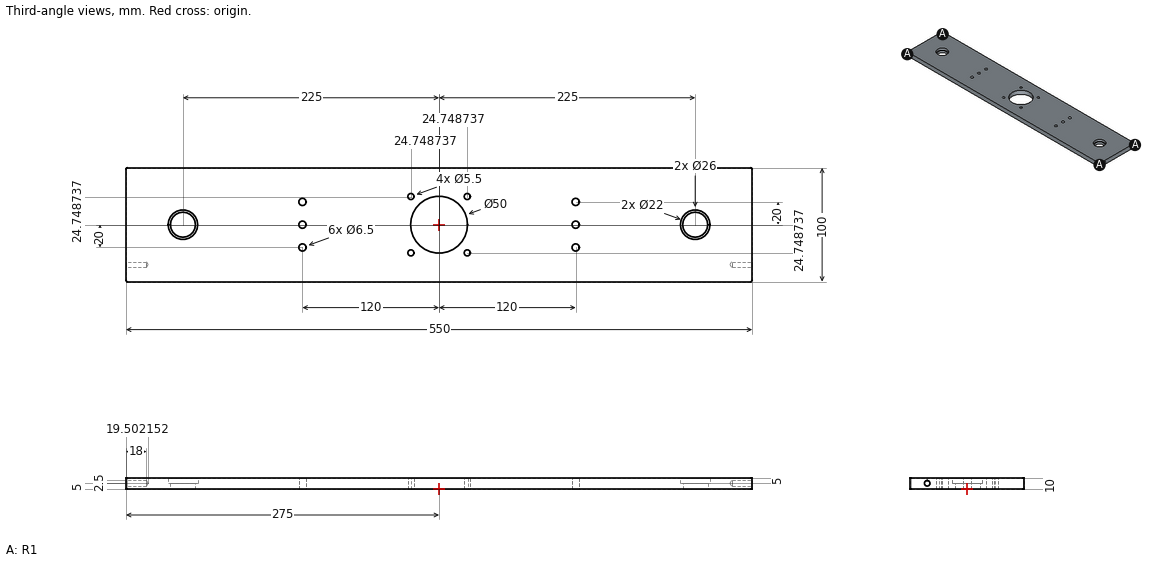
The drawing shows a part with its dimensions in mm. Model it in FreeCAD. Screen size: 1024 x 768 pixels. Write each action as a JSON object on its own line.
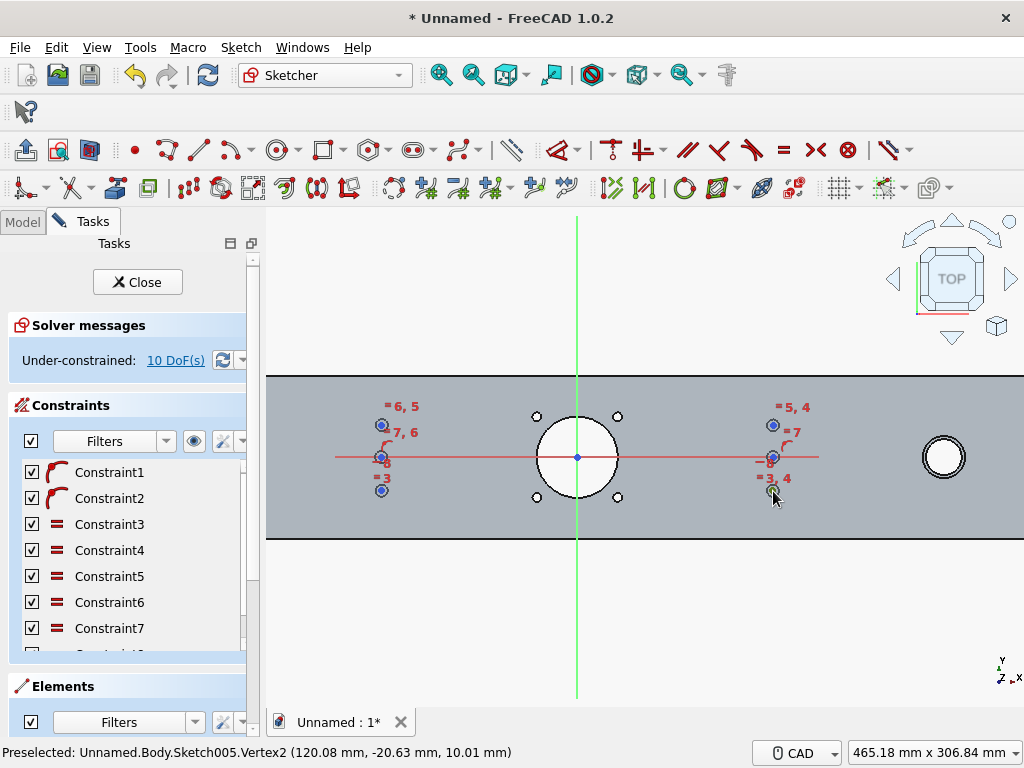
{"action": "left_click", "coordinate": [773, 425]}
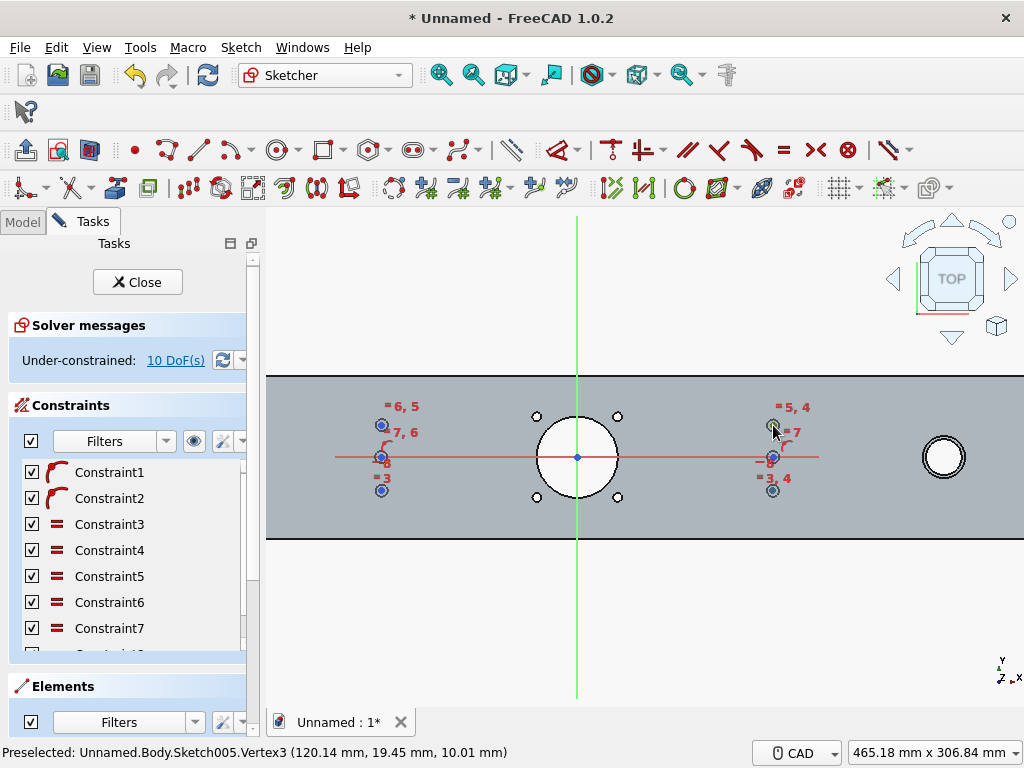
{"action": "left_click", "coordinate": [666, 150]}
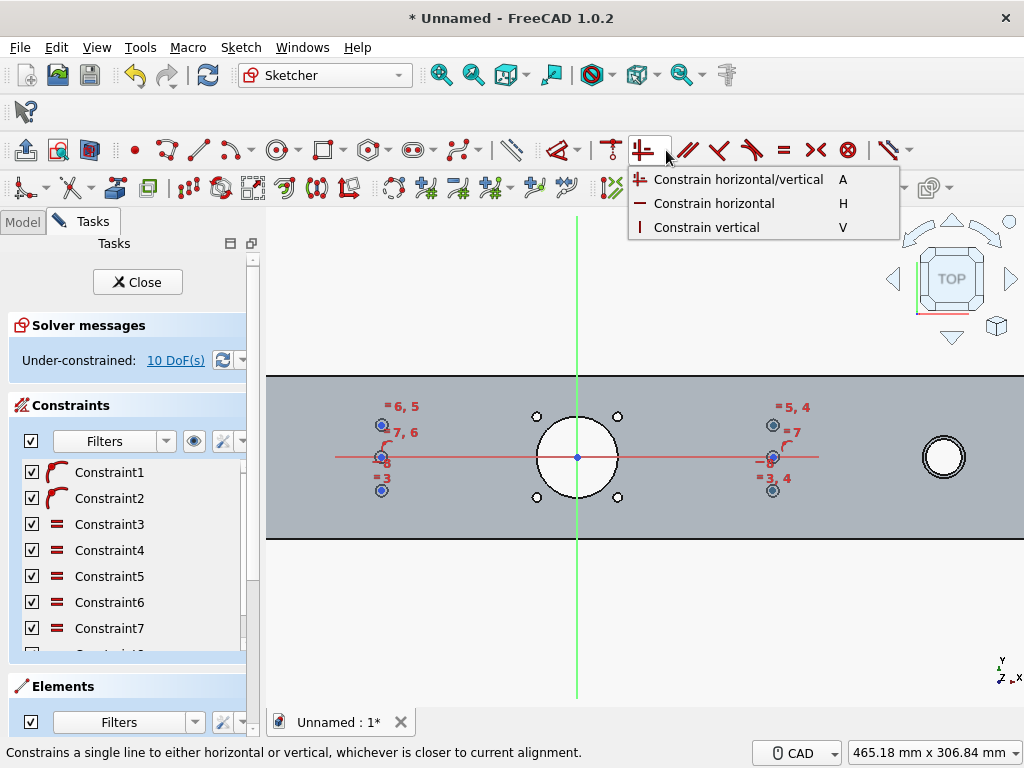
{"action": "left_click", "coordinate": [764, 227]}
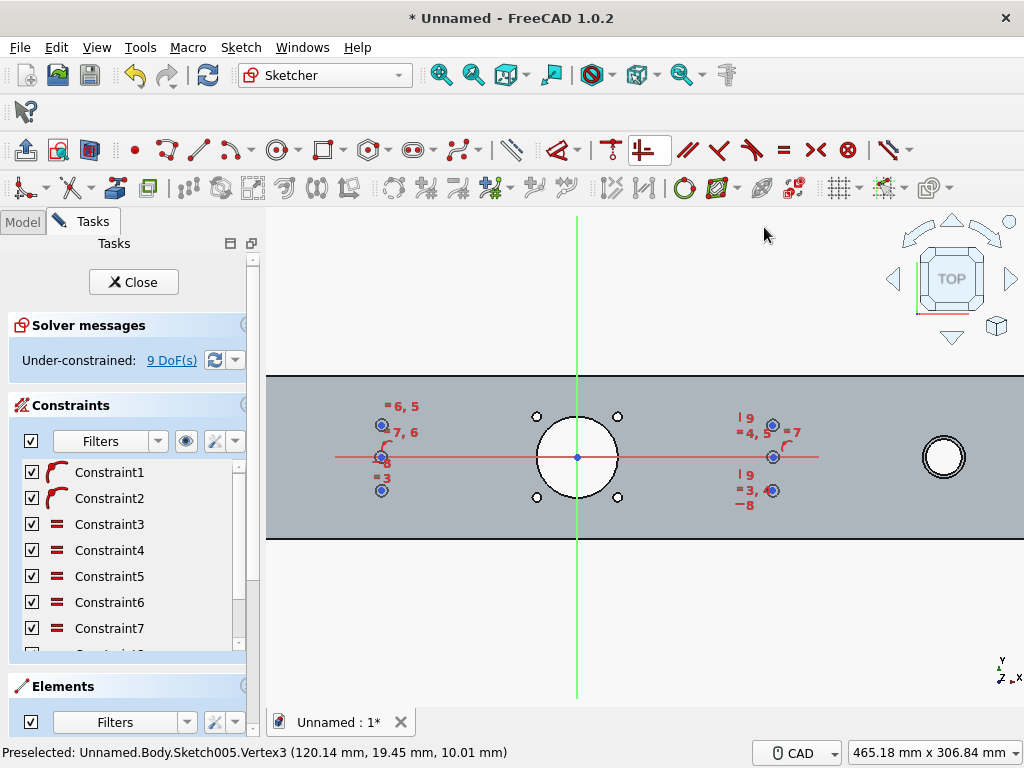
{"action": "left_click", "coordinate": [382, 491]}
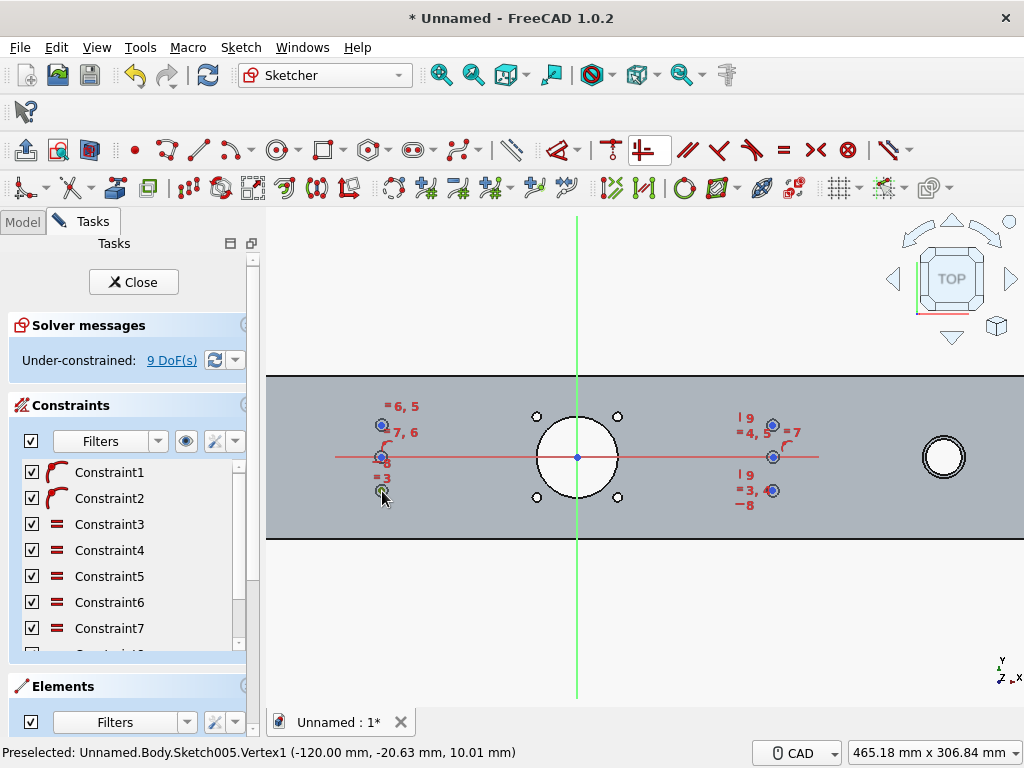
{"action": "left_click", "coordinate": [382, 425]}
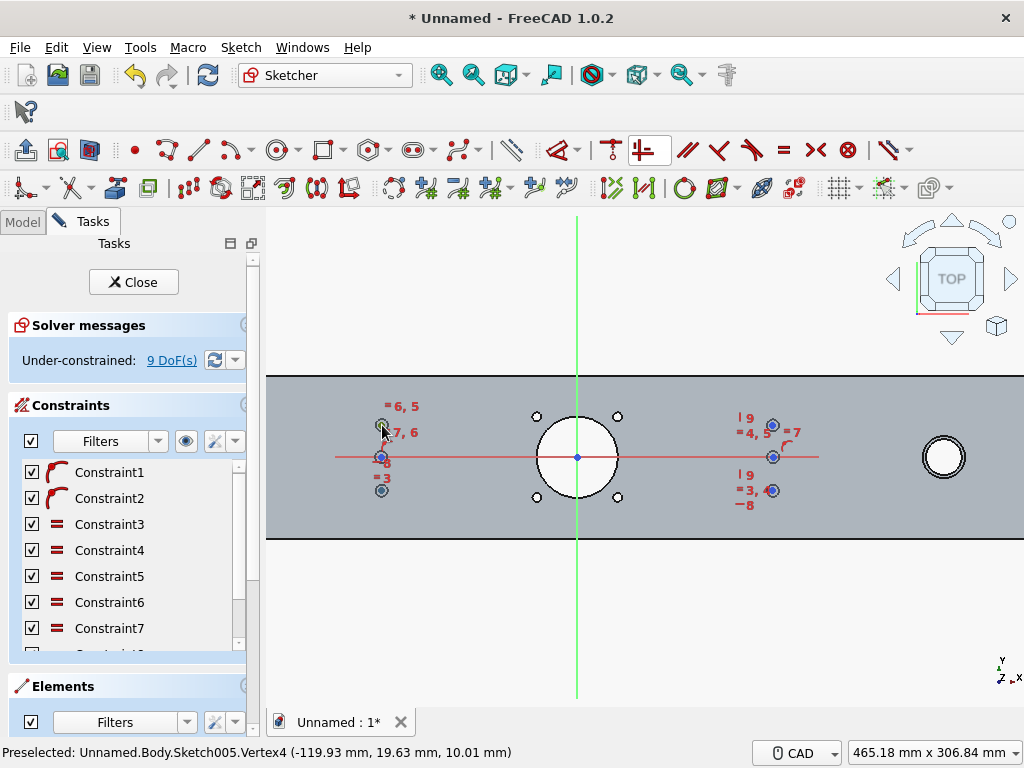
{"action": "key", "text": "v"}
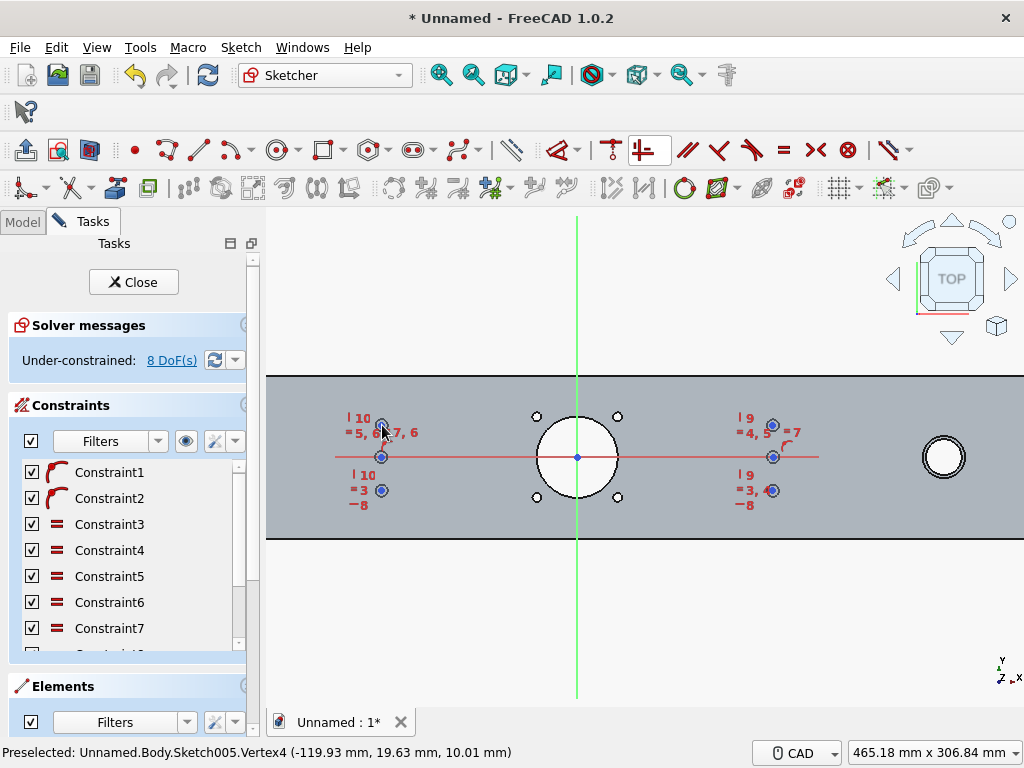
{"action": "left_click", "coordinate": [773, 425]}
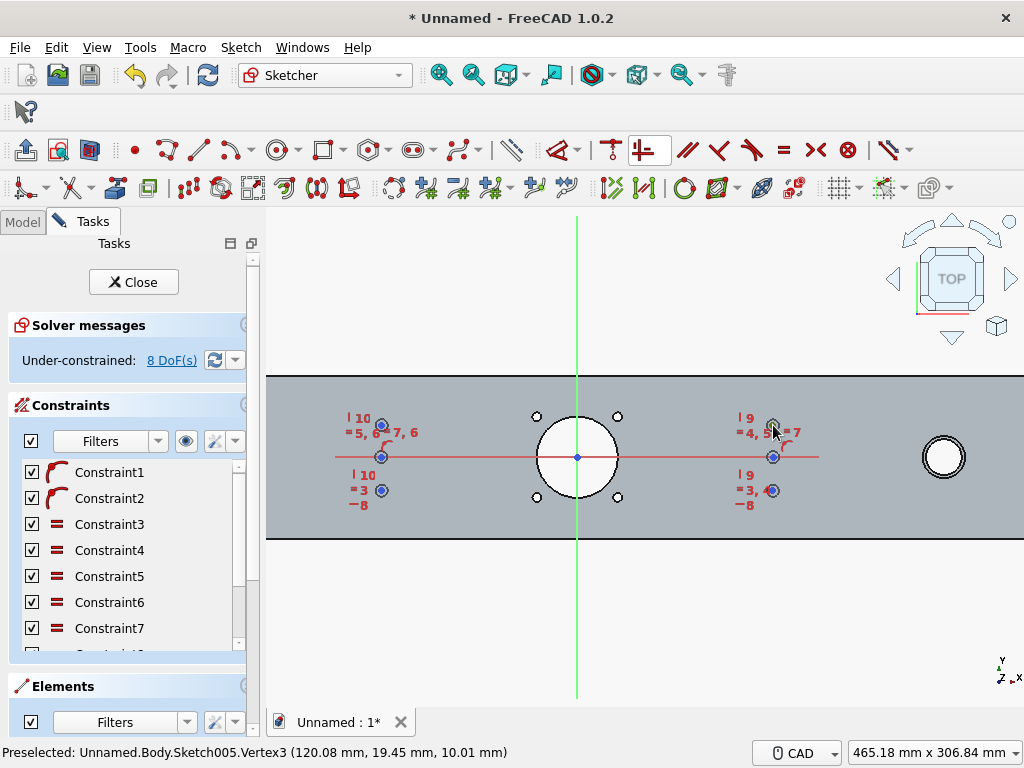
{"action": "left_click", "coordinate": [382, 425]}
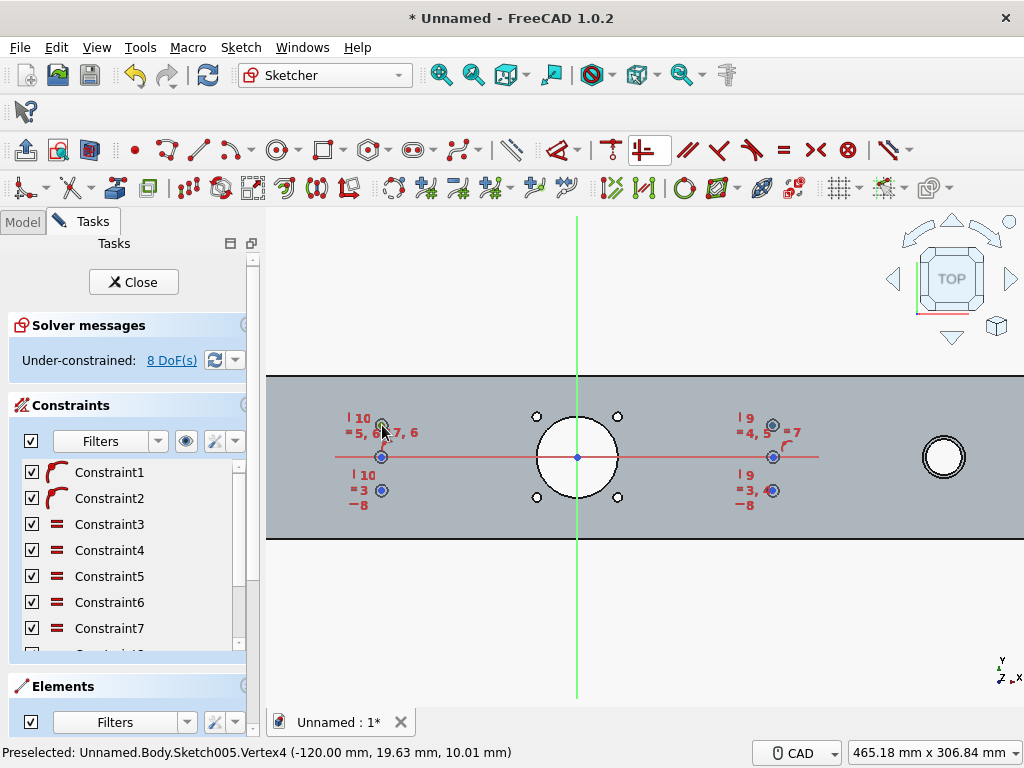
{"action": "key", "text": "h"}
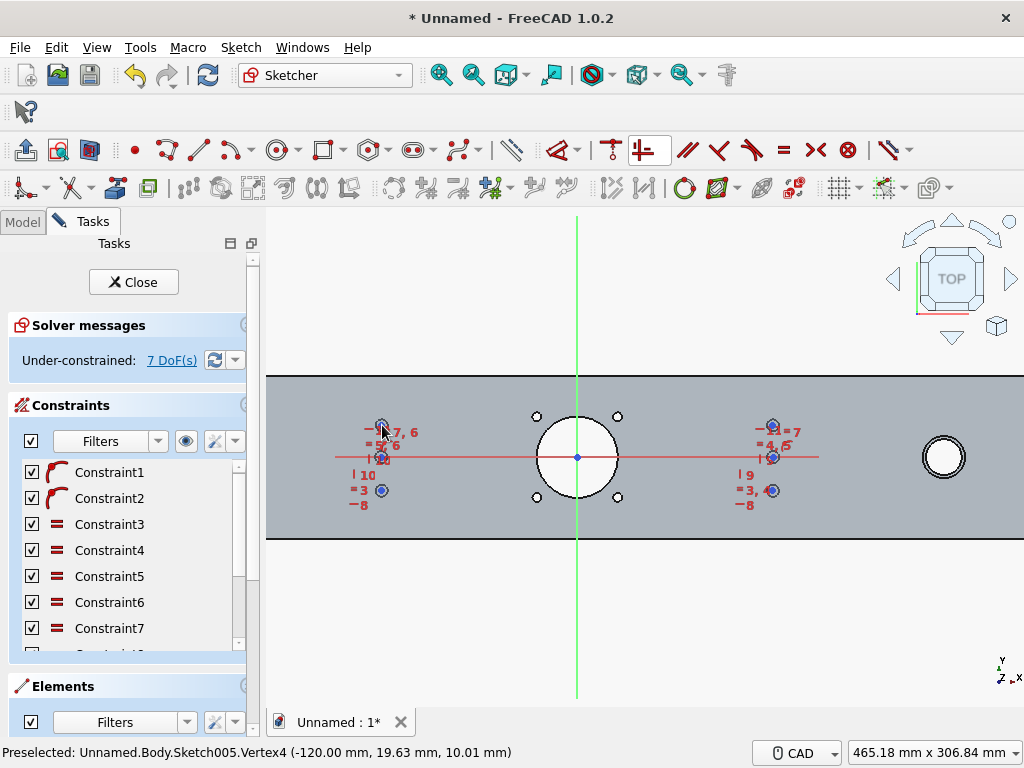
{"action": "left_click", "coordinate": [382, 491]}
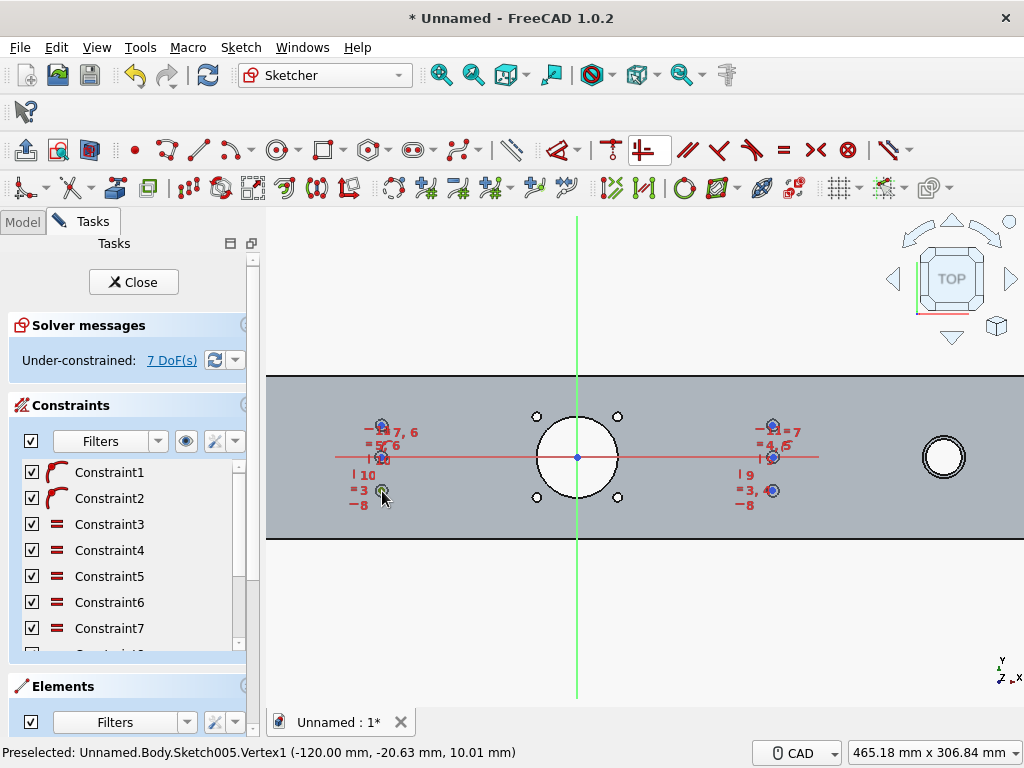
{"action": "scroll", "coordinate": [381, 457], "scroll_direction": "up", "scroll_amount": 4}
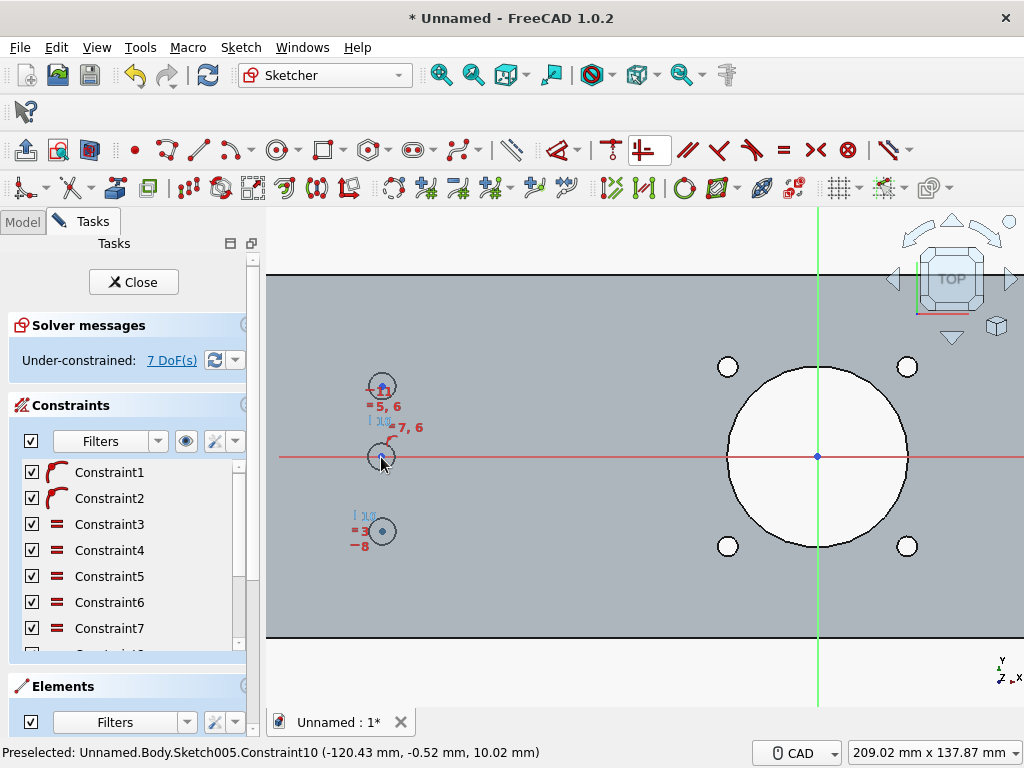
{"action": "left_click", "coordinate": [381, 457]}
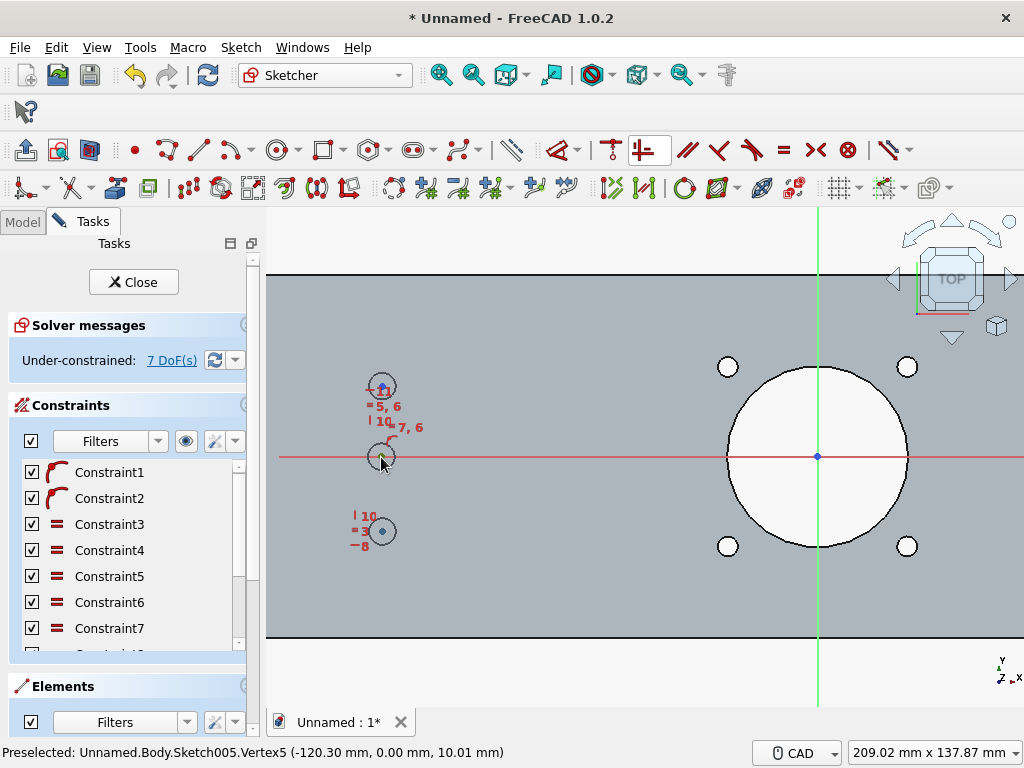
{"action": "left_click", "coordinate": [666, 150]}